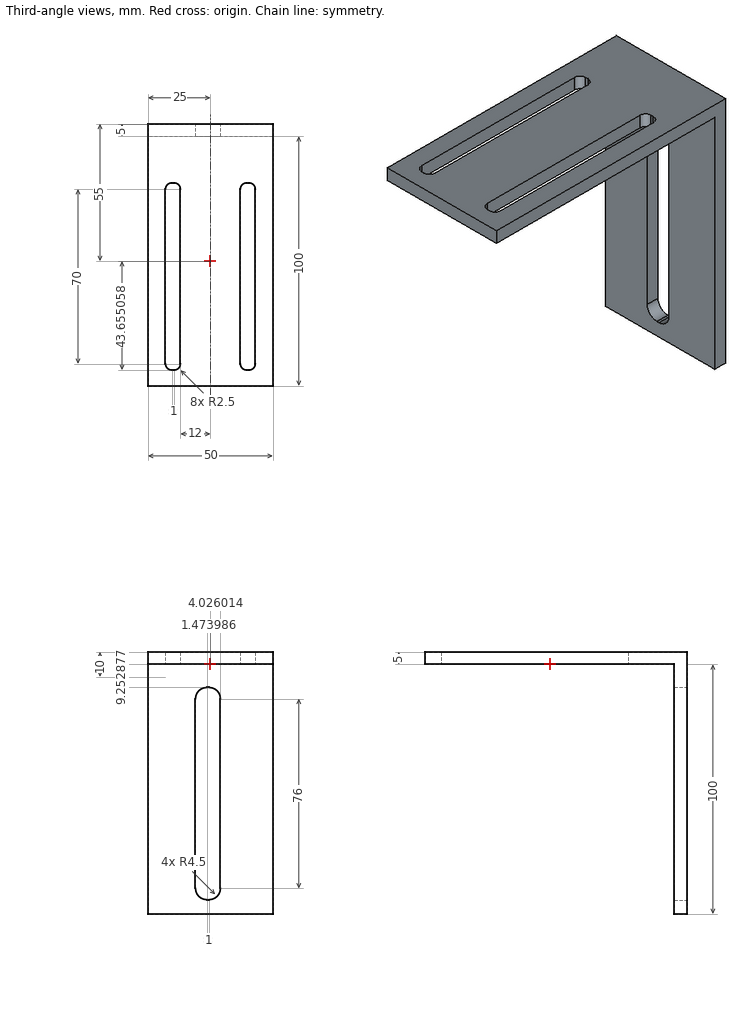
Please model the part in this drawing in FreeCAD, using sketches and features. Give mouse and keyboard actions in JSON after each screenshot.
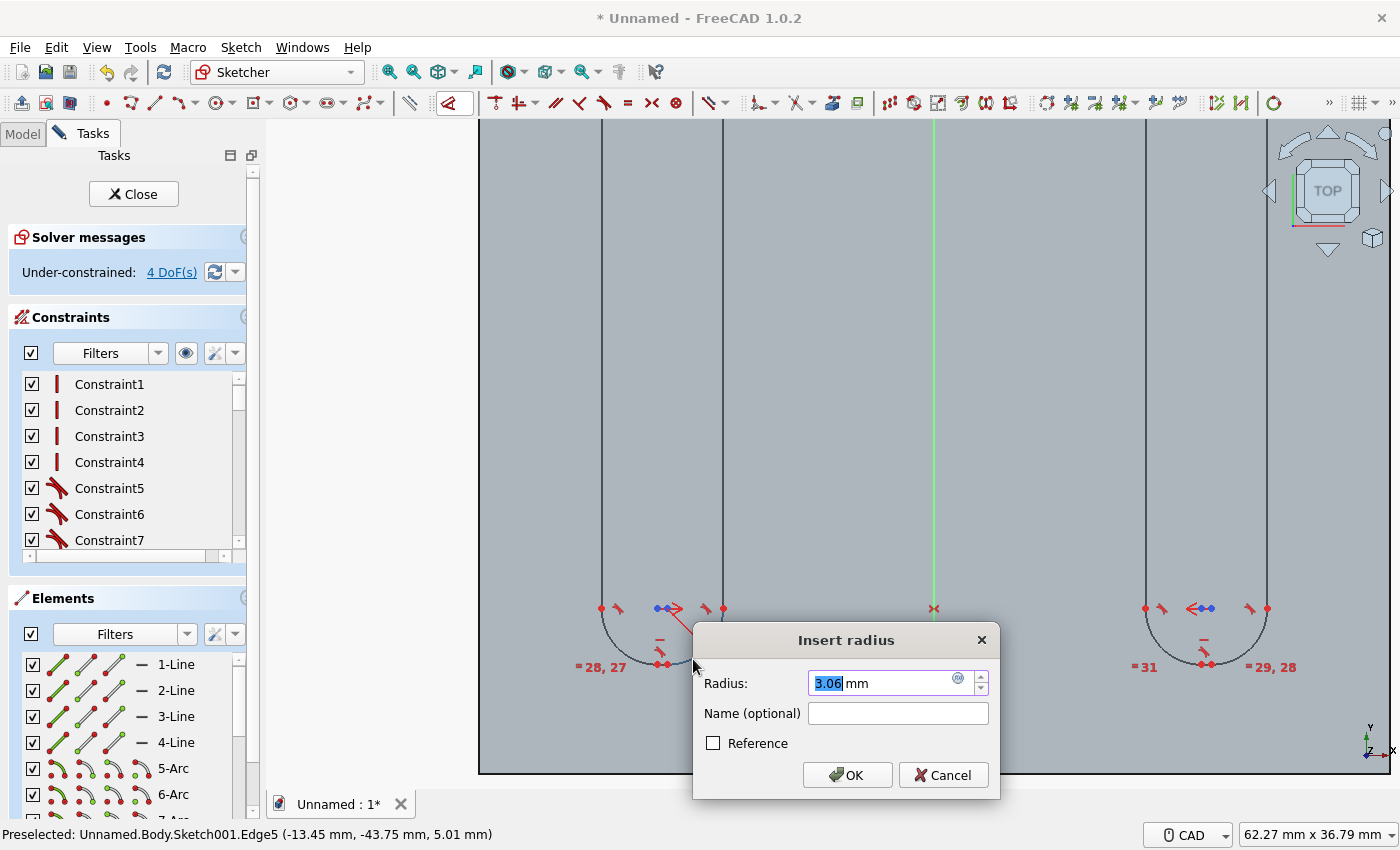
{"action": "type", "text": "2.5"}
{"action": "key", "text": "Return"}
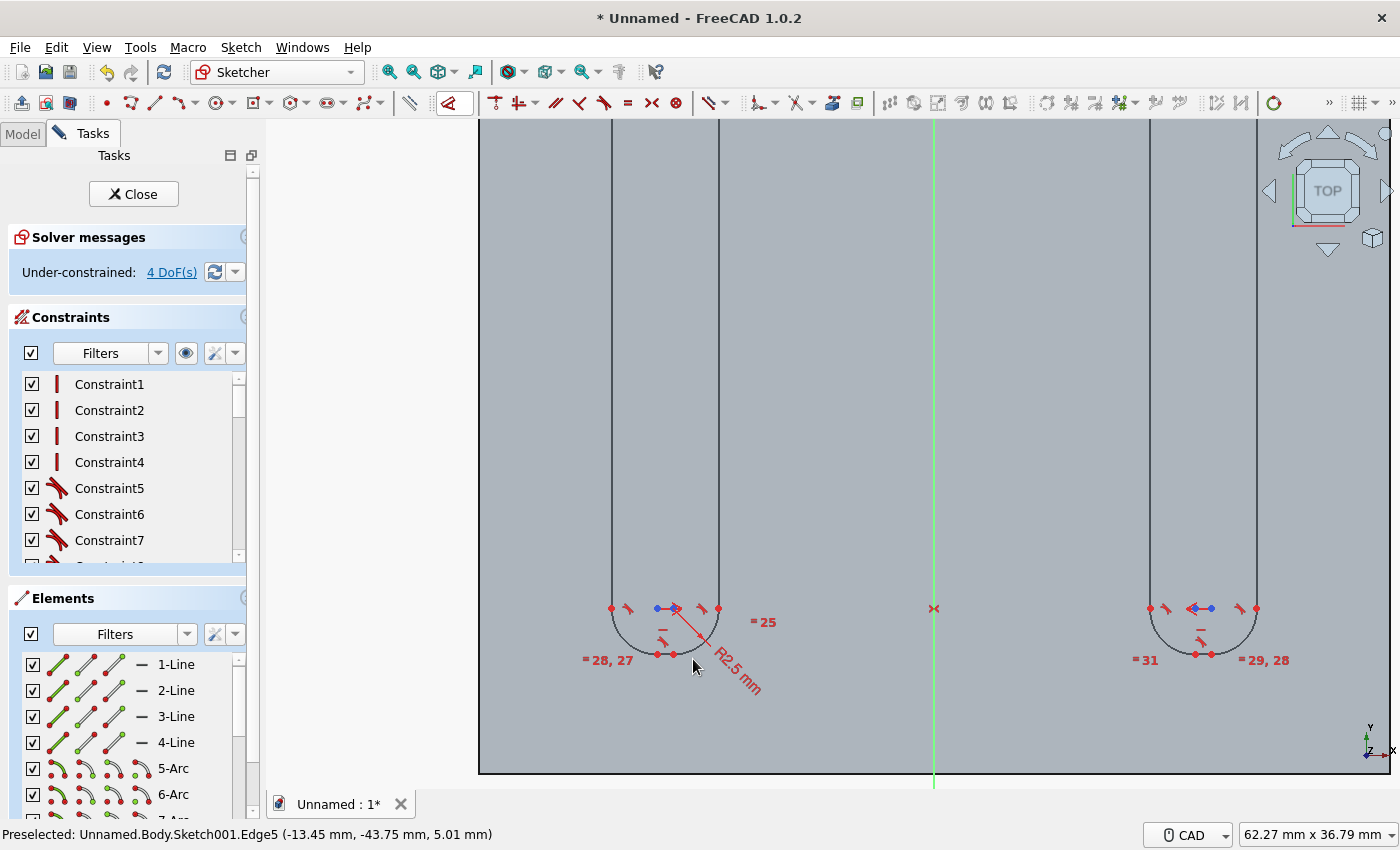
{"action": "scroll", "coordinate": [665, 654], "scroll_direction": "up", "scroll_amount": 4}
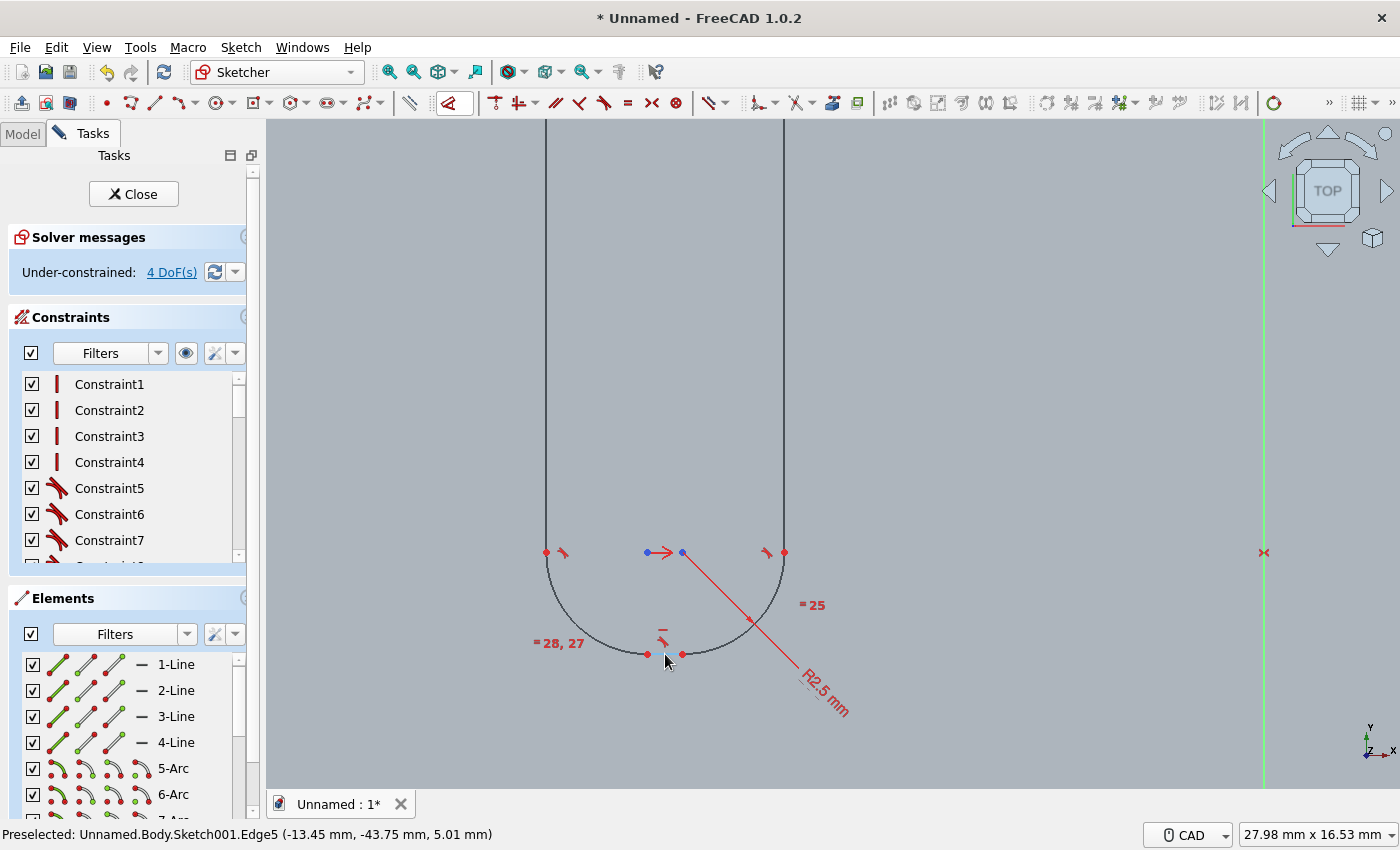
{"action": "left_click", "coordinate": [665, 654]}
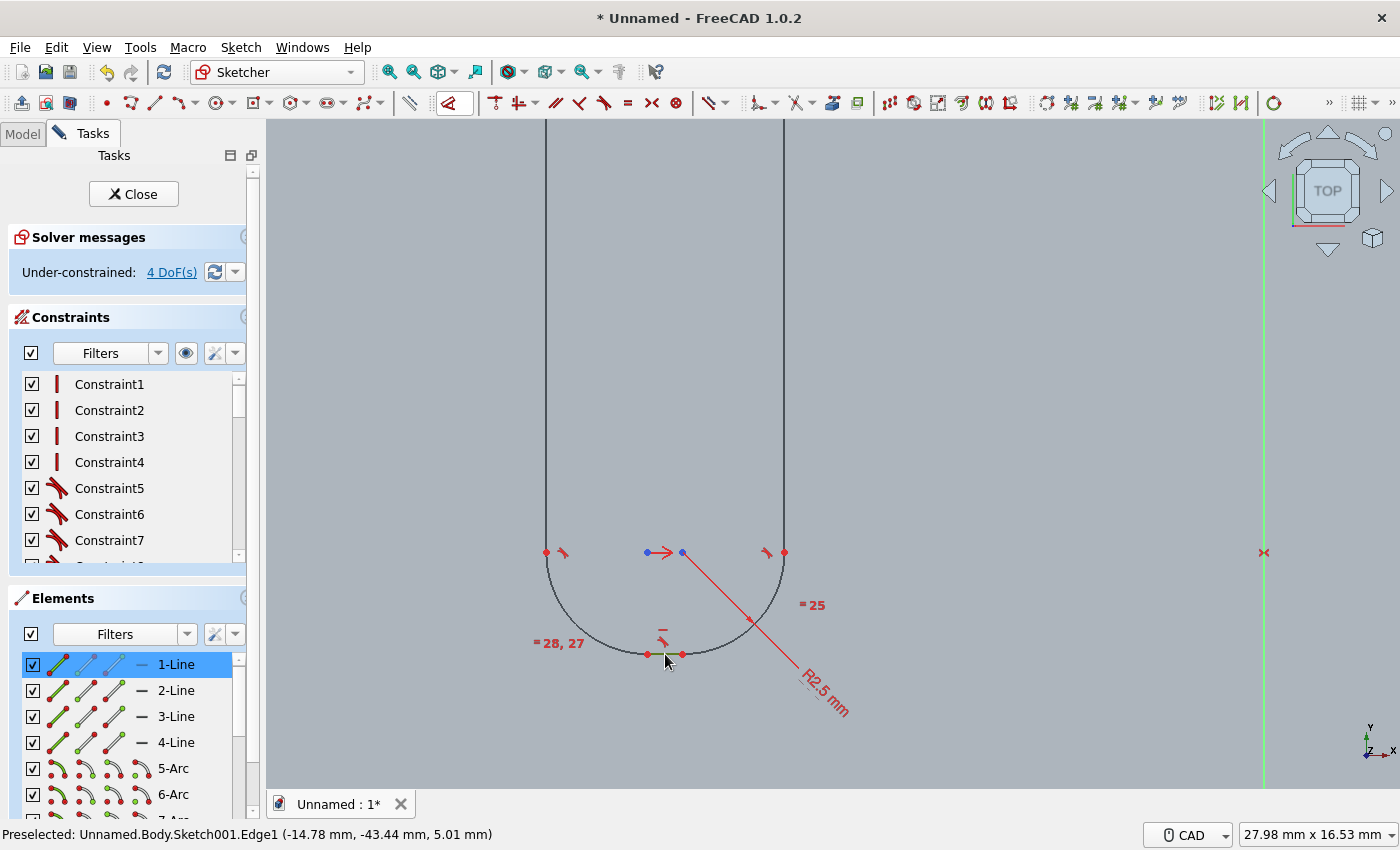
{"action": "key", "text": "l"}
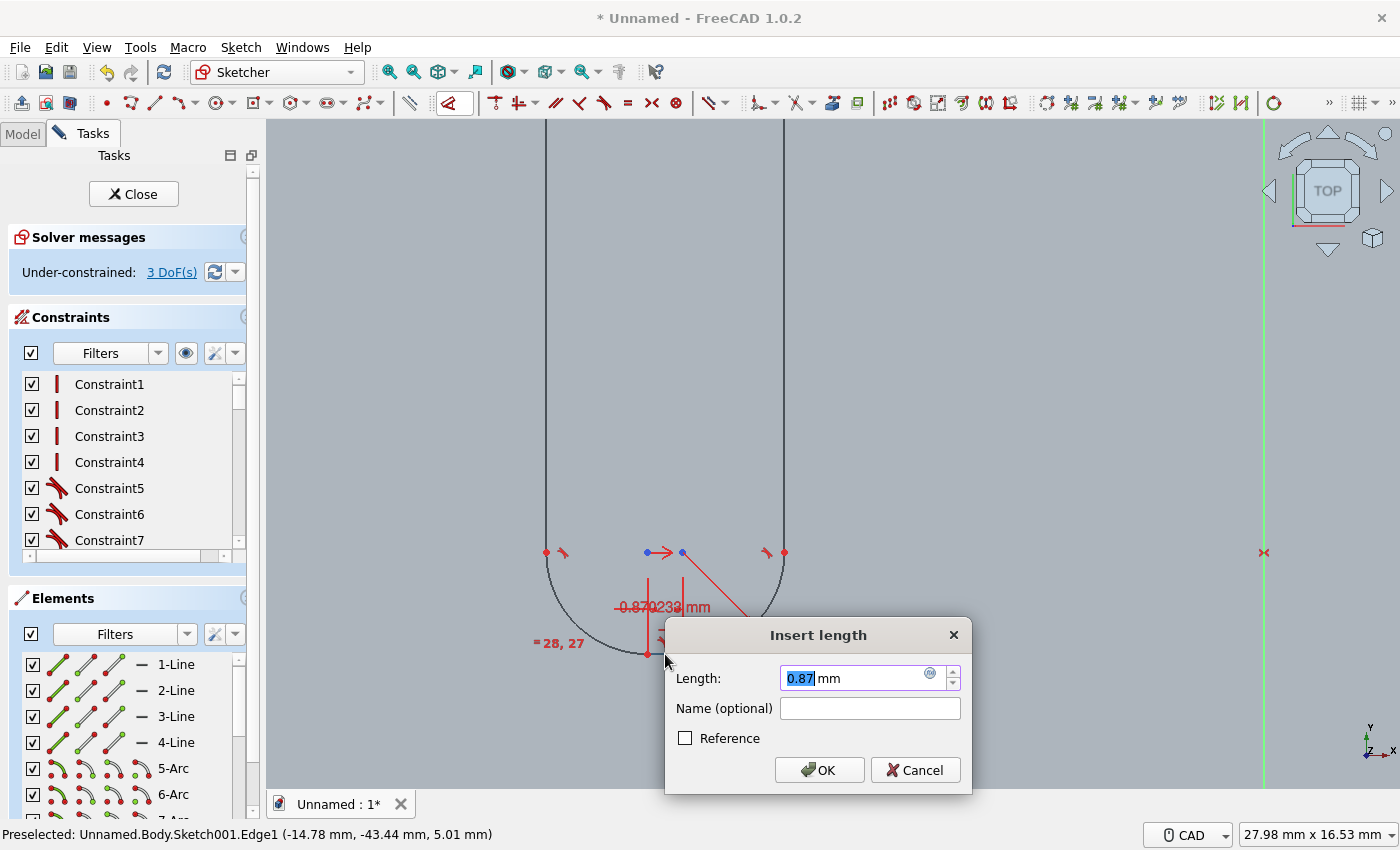
{"action": "type", "text": "1"}
{"action": "key", "text": "Return"}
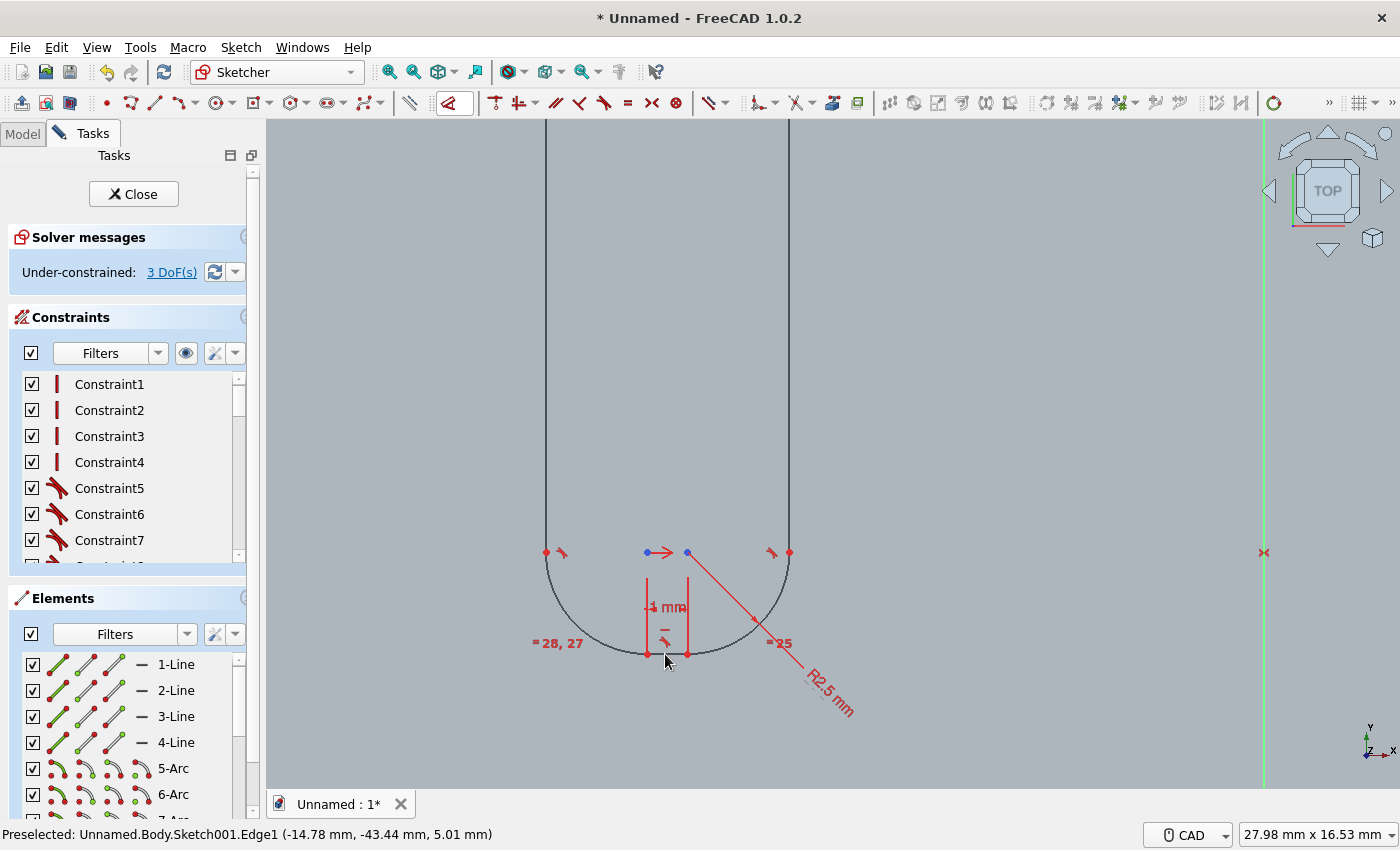
{"action": "scroll", "coordinate": [686, 659], "scroll_direction": "down", "scroll_amount": 10}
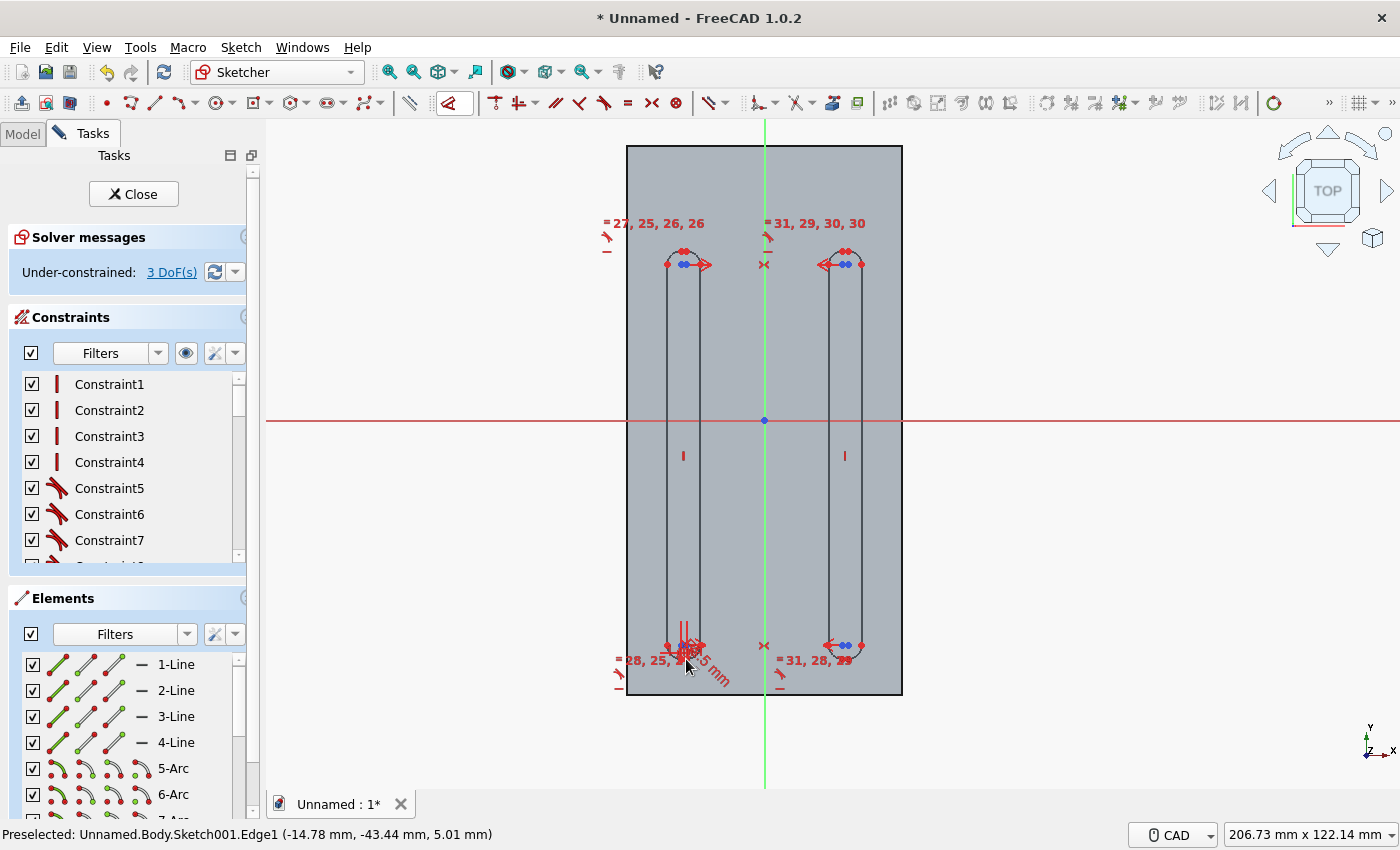
{"action": "left_click", "coordinate": [700, 531]}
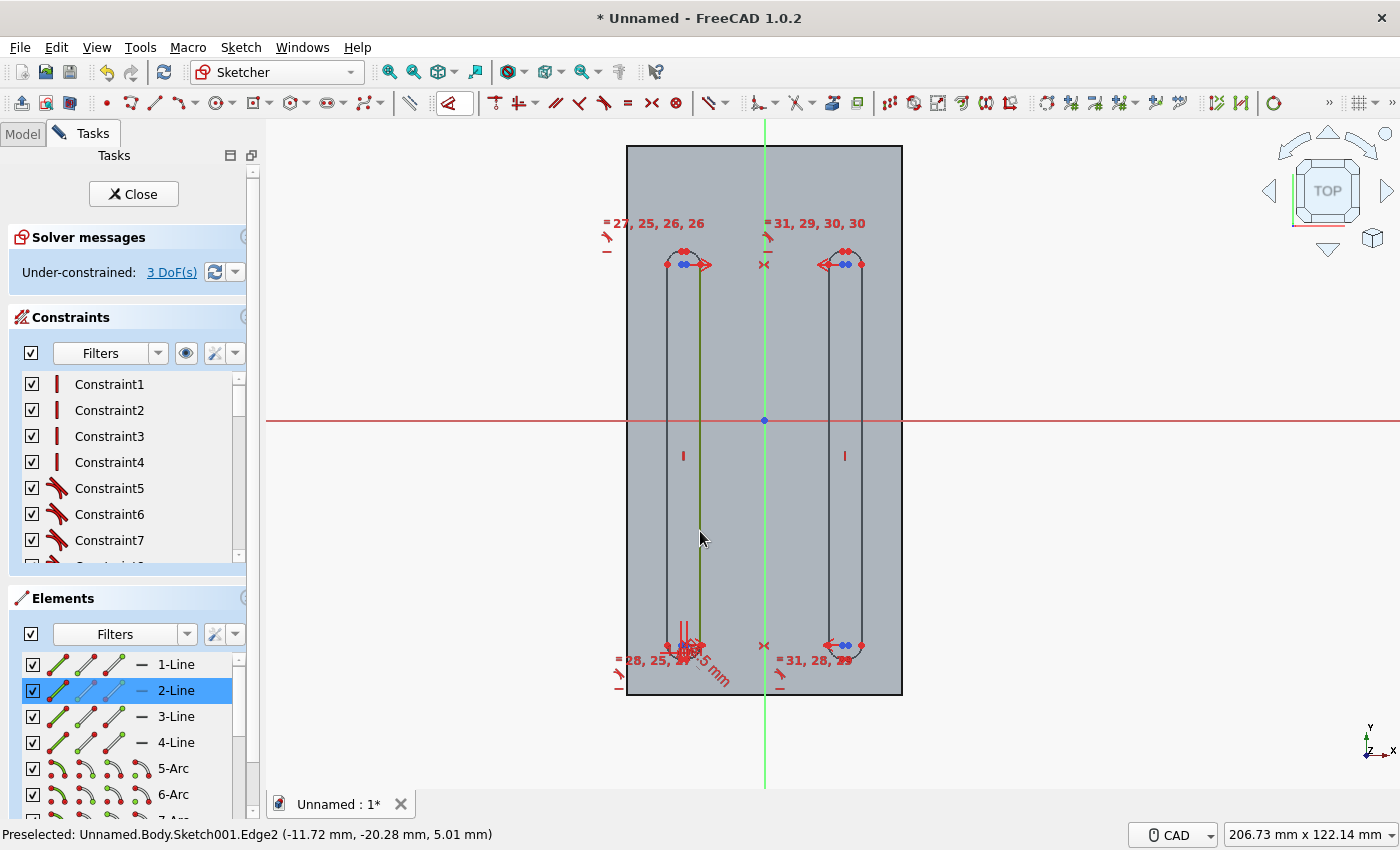
{"action": "key", "text": "i"}